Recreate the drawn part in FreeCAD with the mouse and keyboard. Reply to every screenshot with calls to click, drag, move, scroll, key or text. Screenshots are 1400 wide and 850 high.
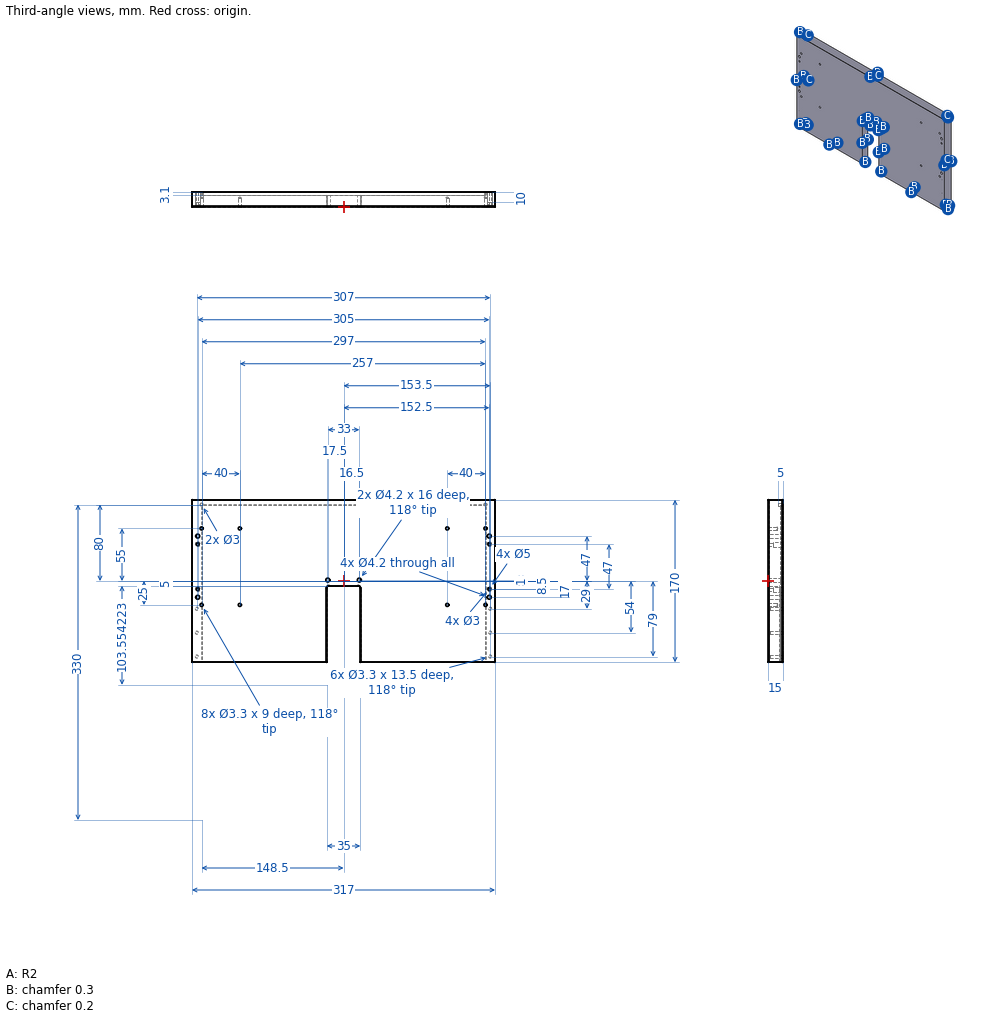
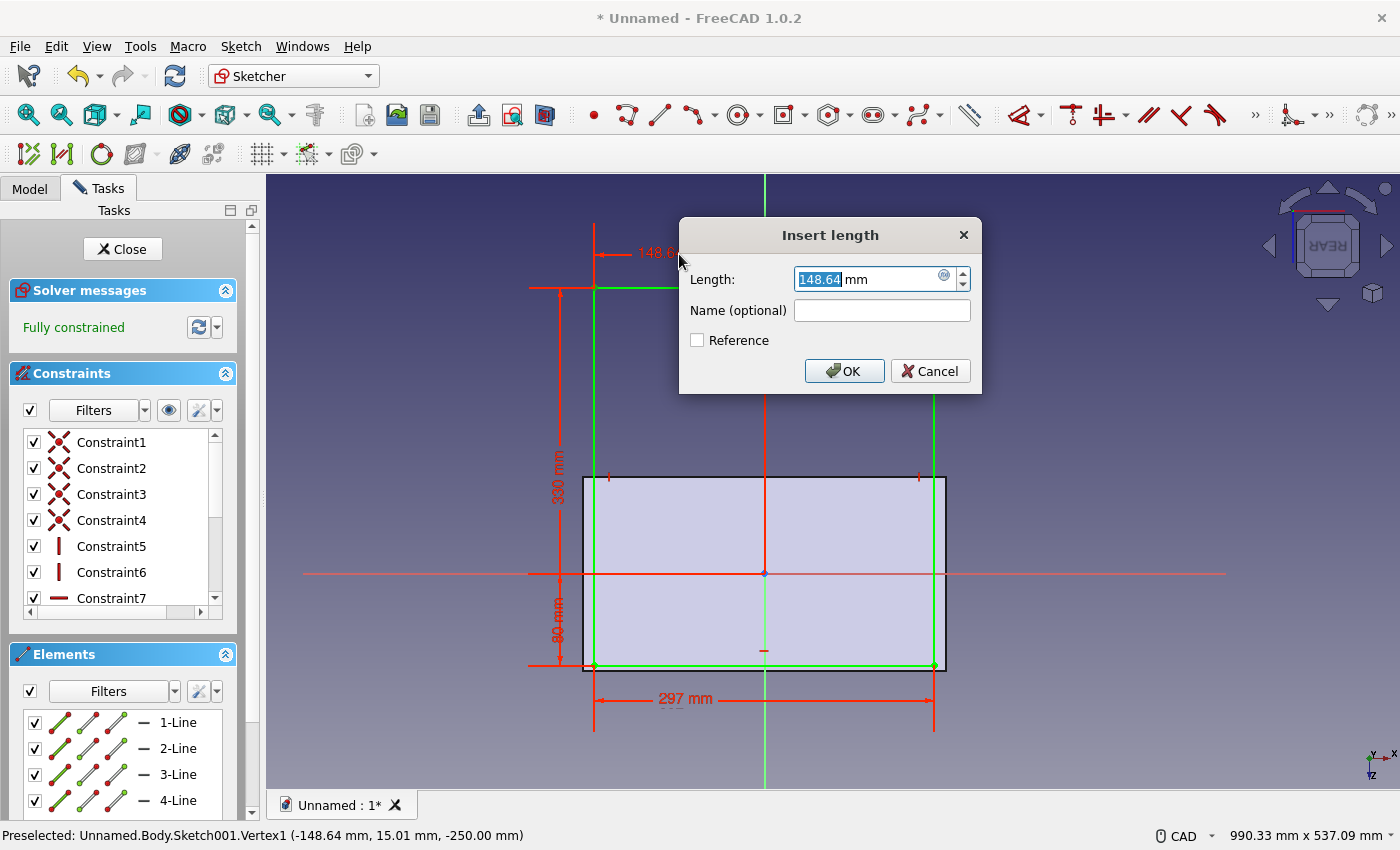
text(148.5)
key(Return)
key(Escape)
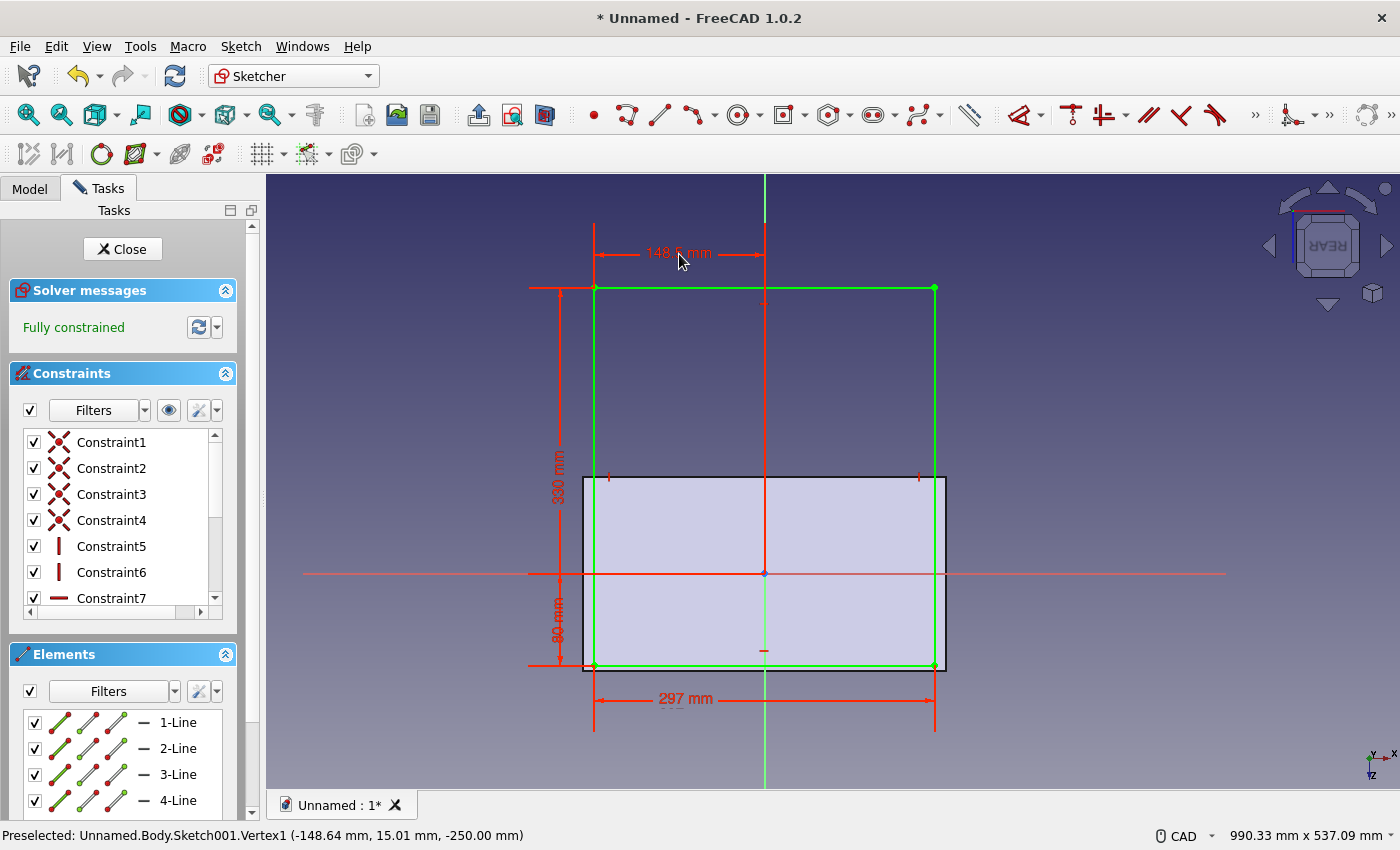
click(123, 249)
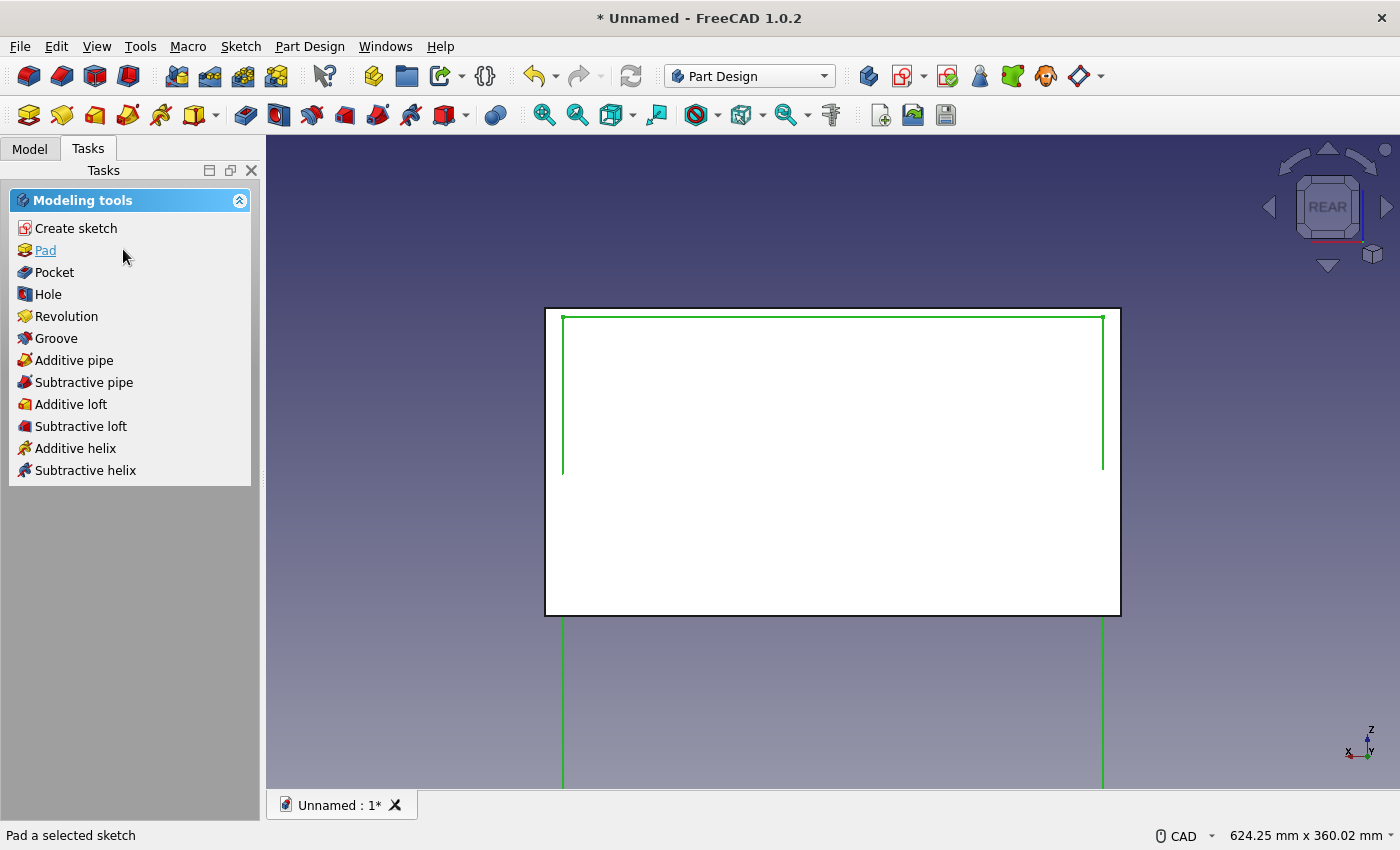
click(246, 116)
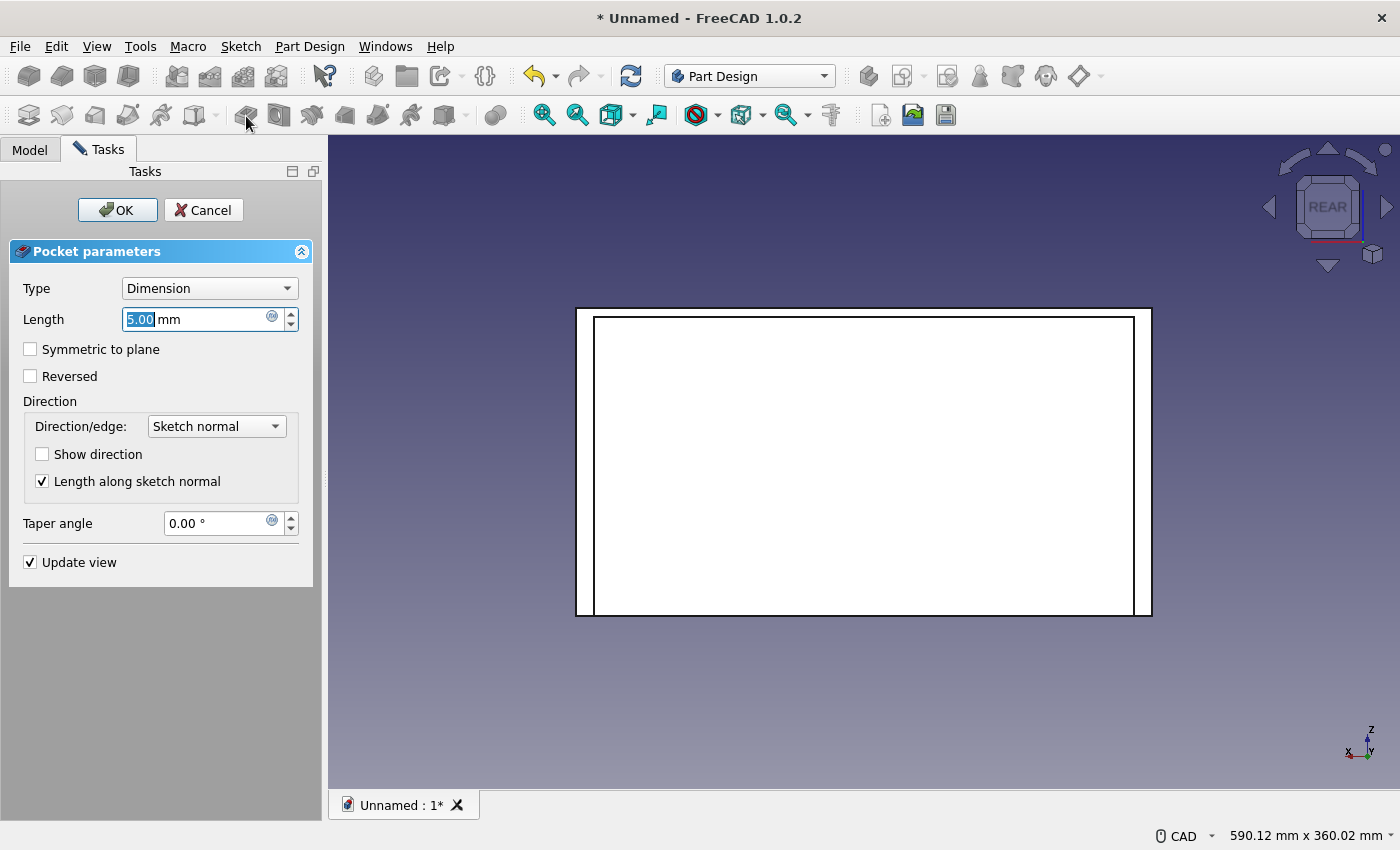
text(3.1)
key(Tab)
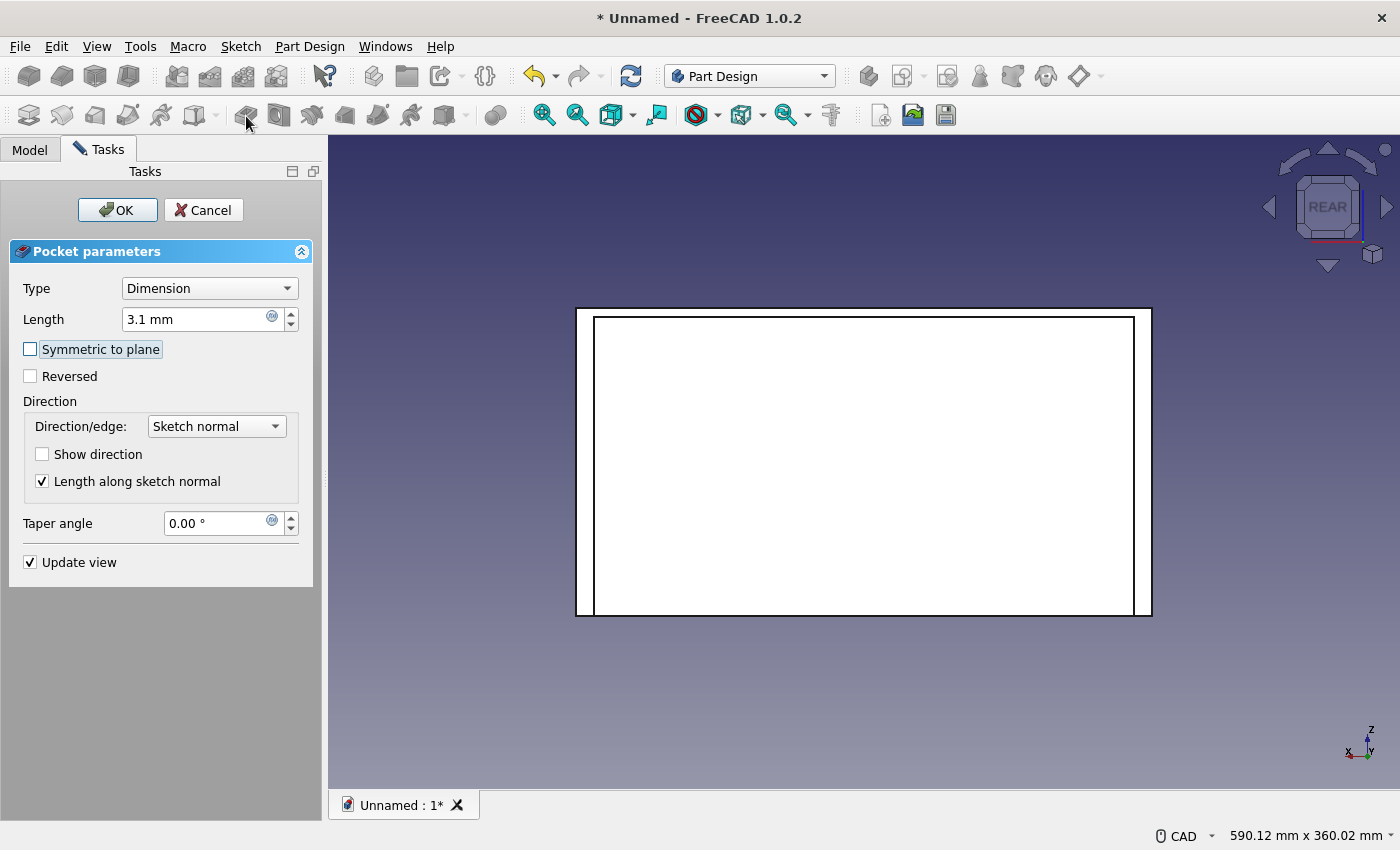
click(118, 210)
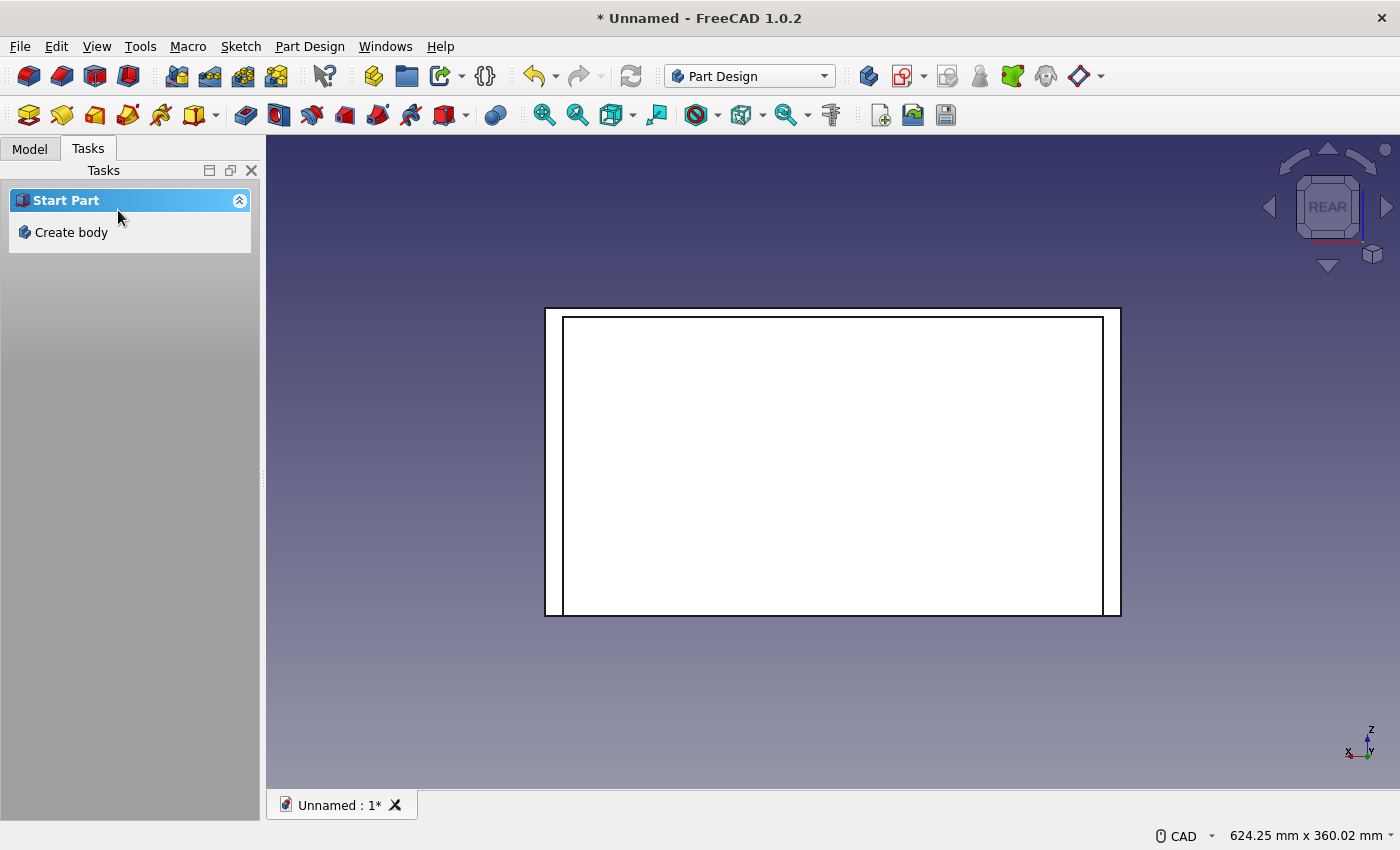
key(0)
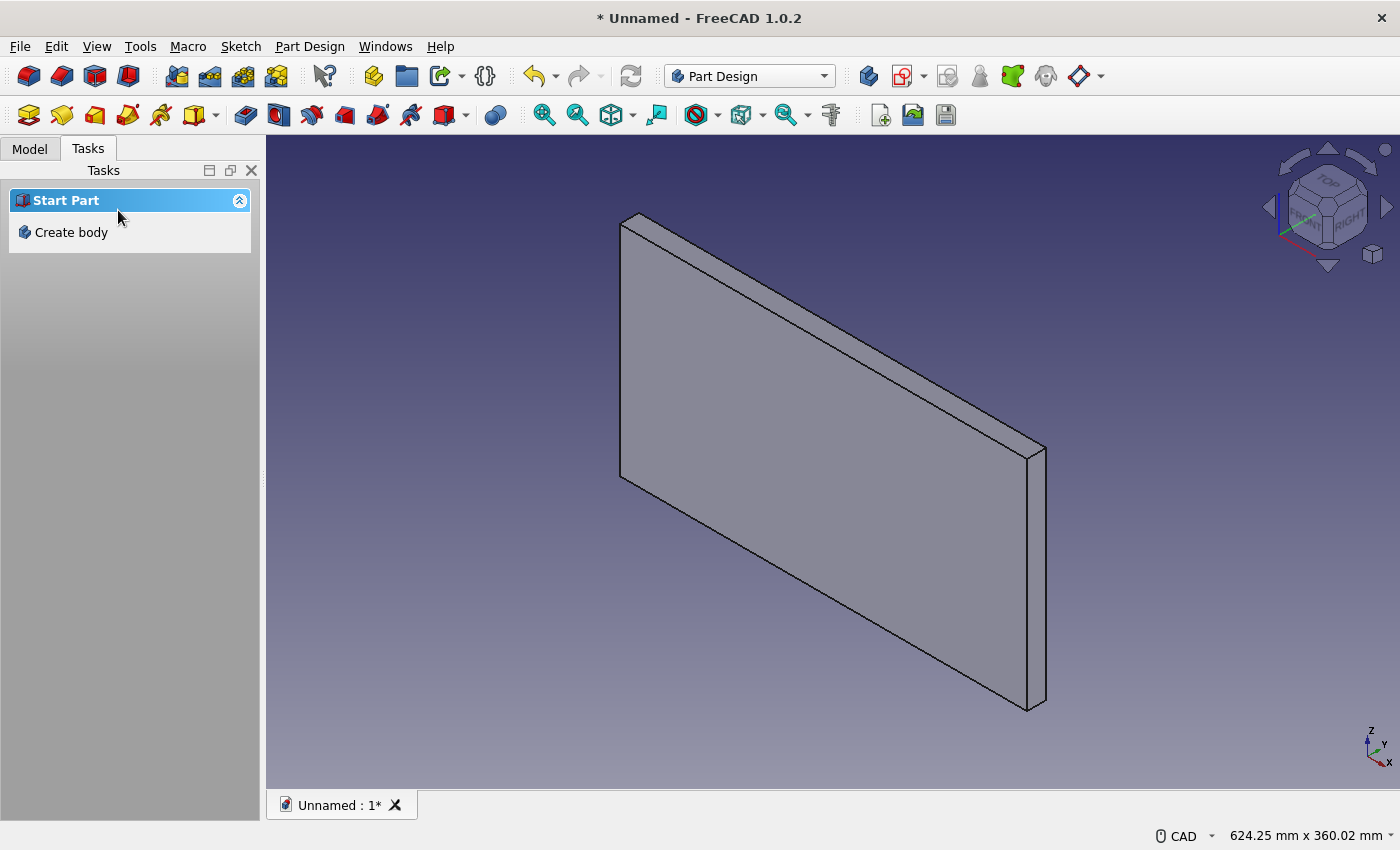
click(882, 500)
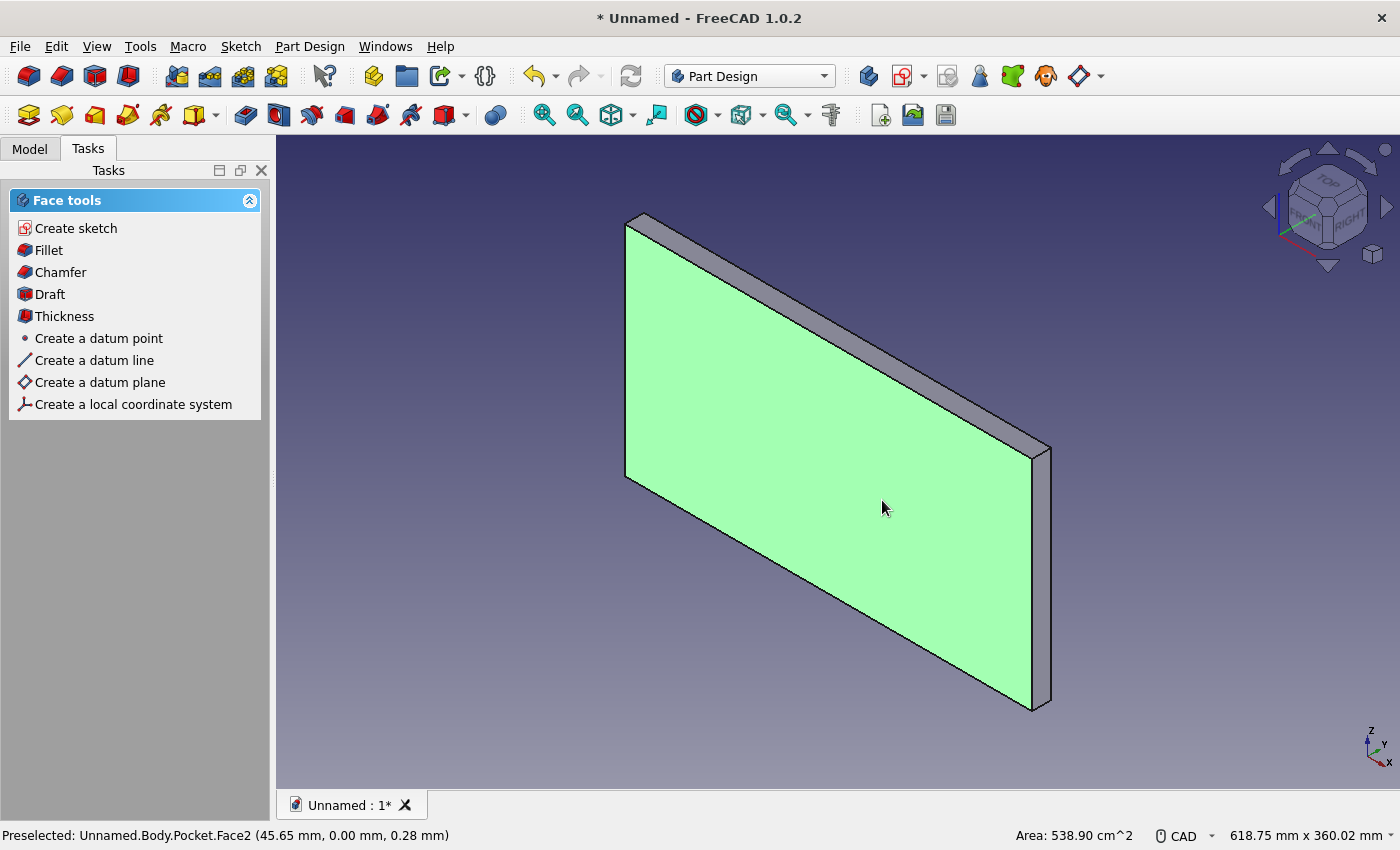
click(902, 76)